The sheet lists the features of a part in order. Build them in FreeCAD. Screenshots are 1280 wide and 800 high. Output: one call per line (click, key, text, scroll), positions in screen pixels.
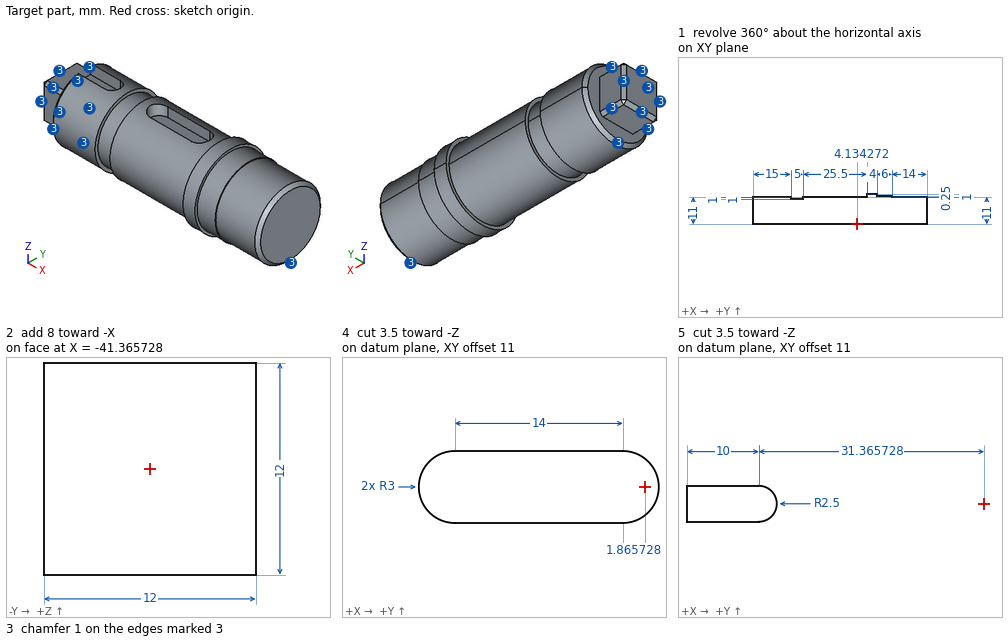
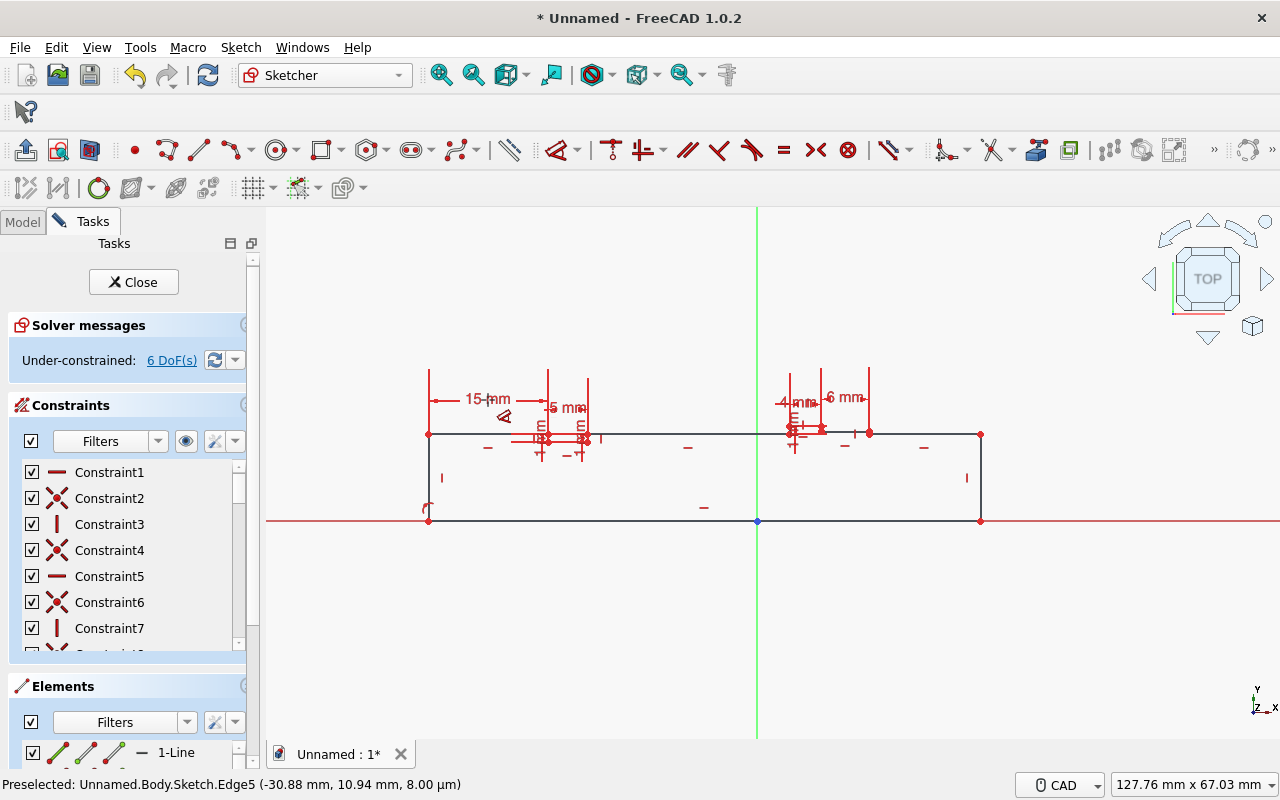
click(429, 460)
click(395, 478)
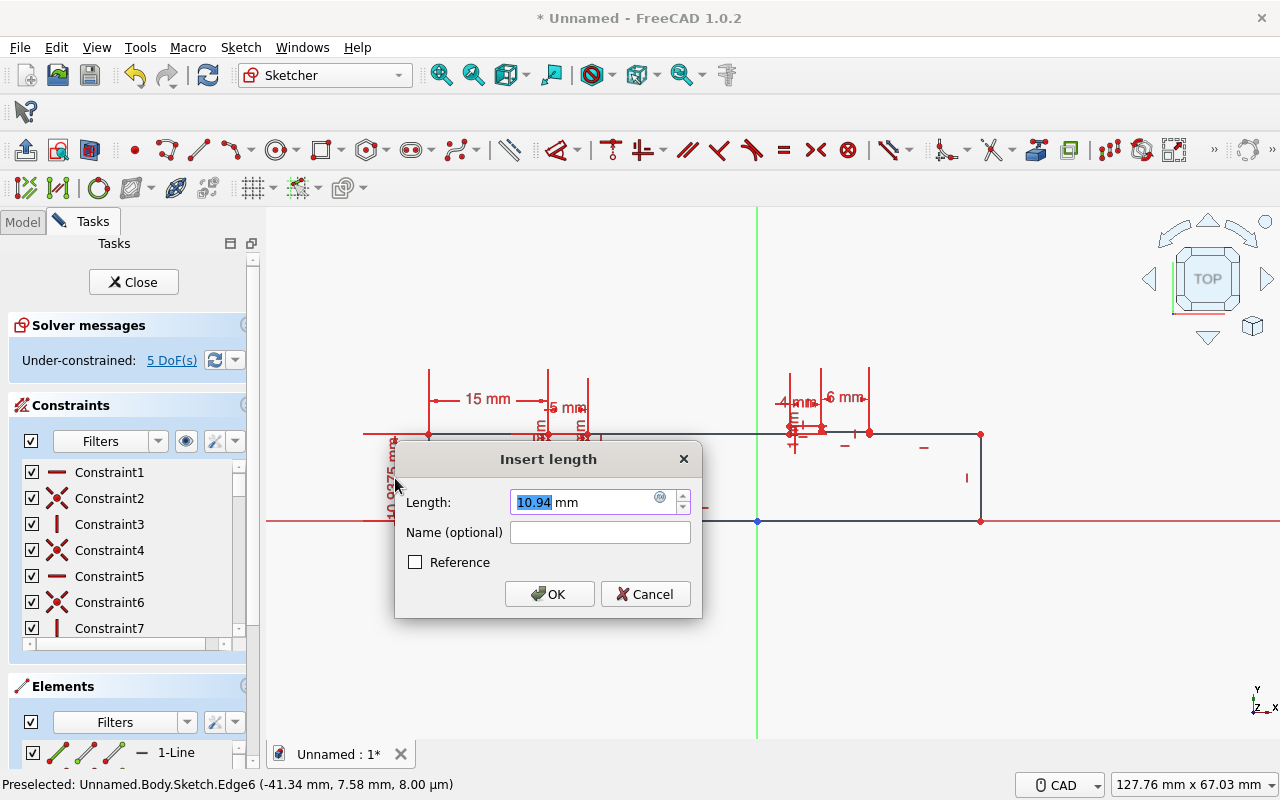
text(11)
key(Return)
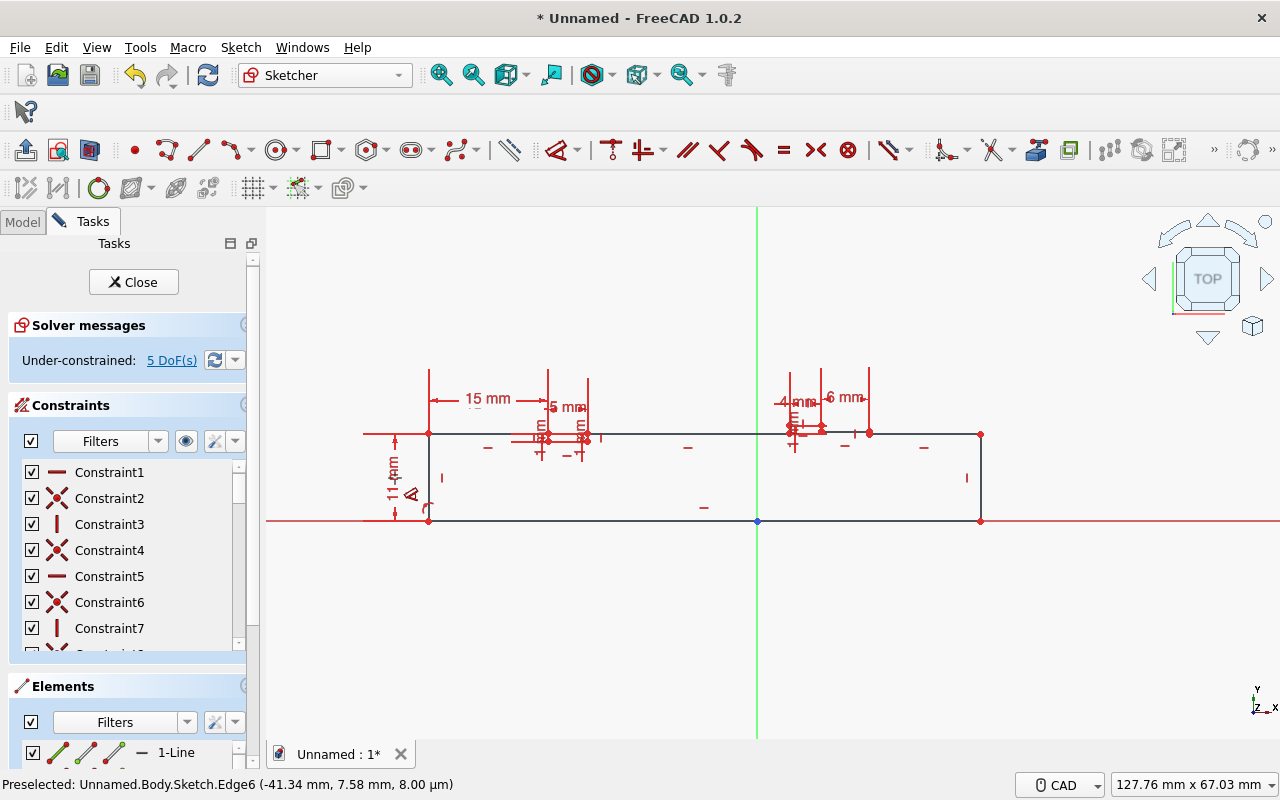
click(981, 495)
click(1015, 478)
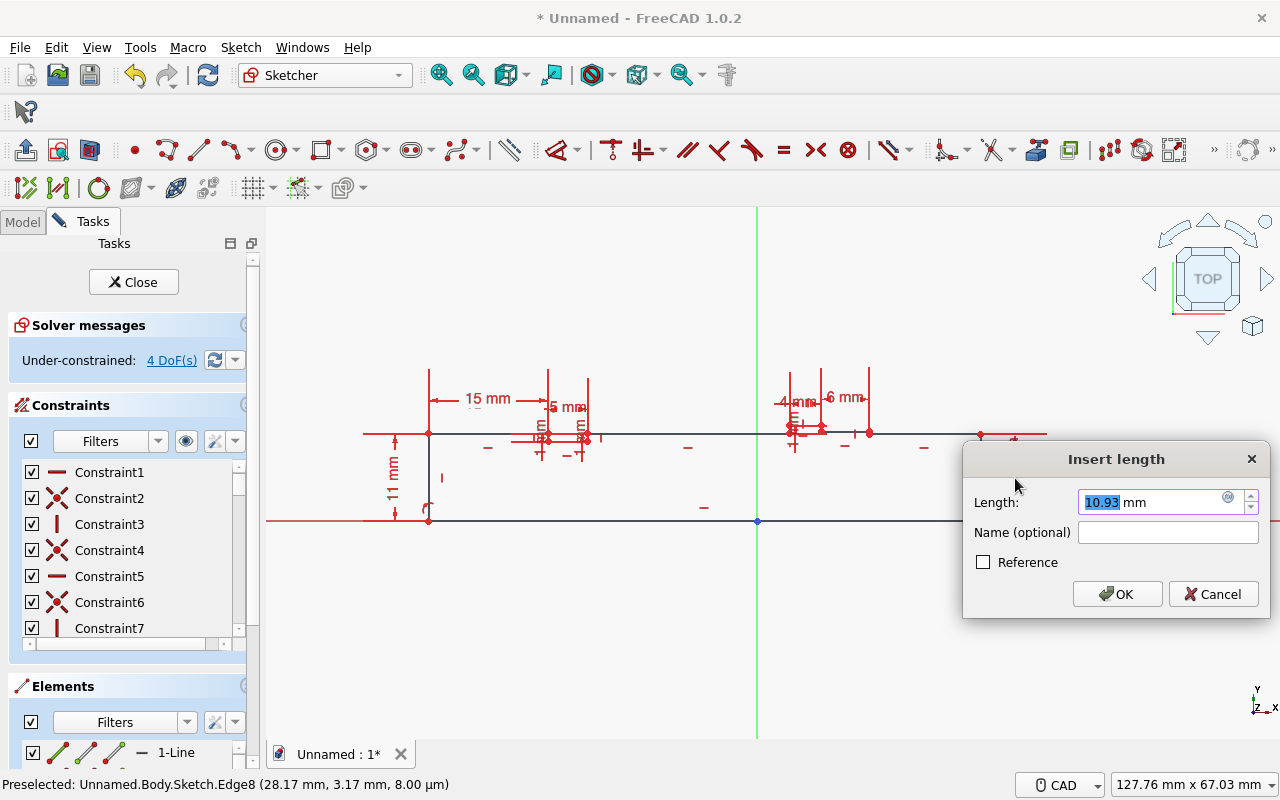
text(11)
key(Return)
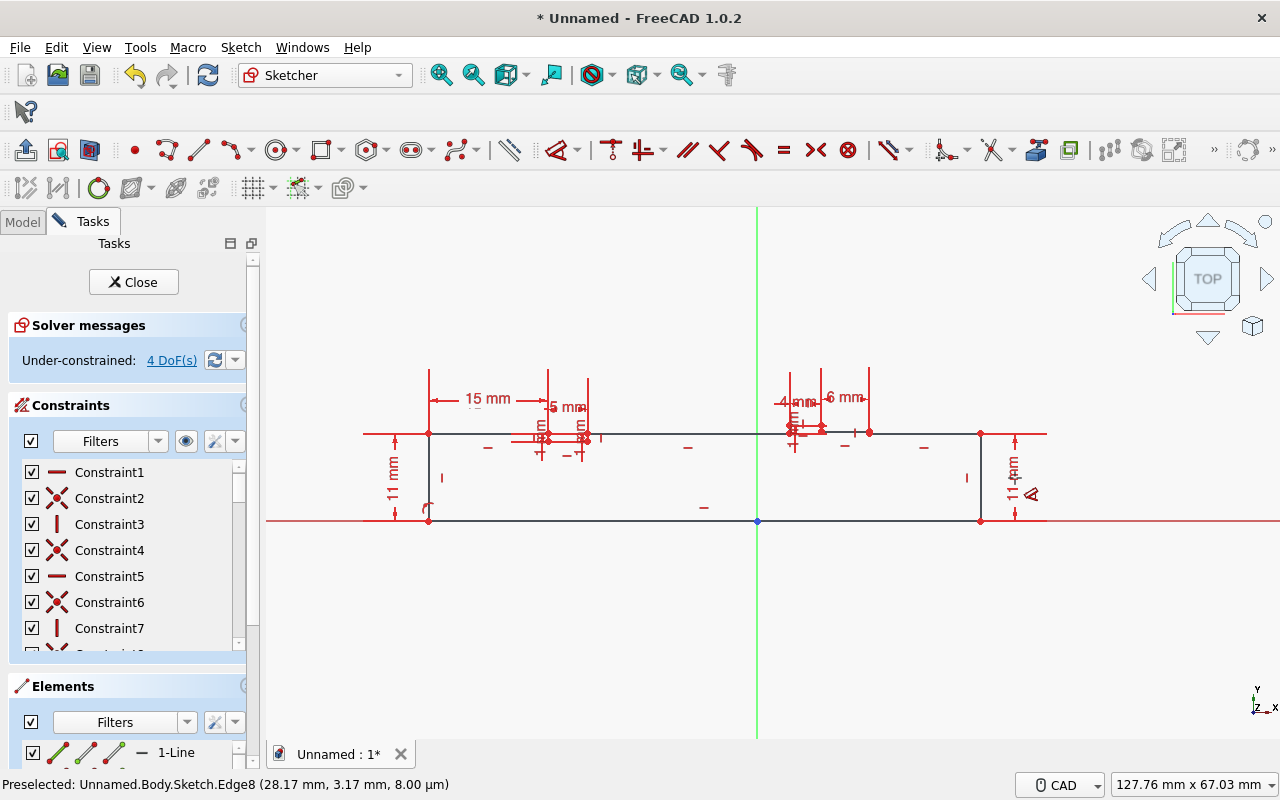
click(947, 434)
click(925, 400)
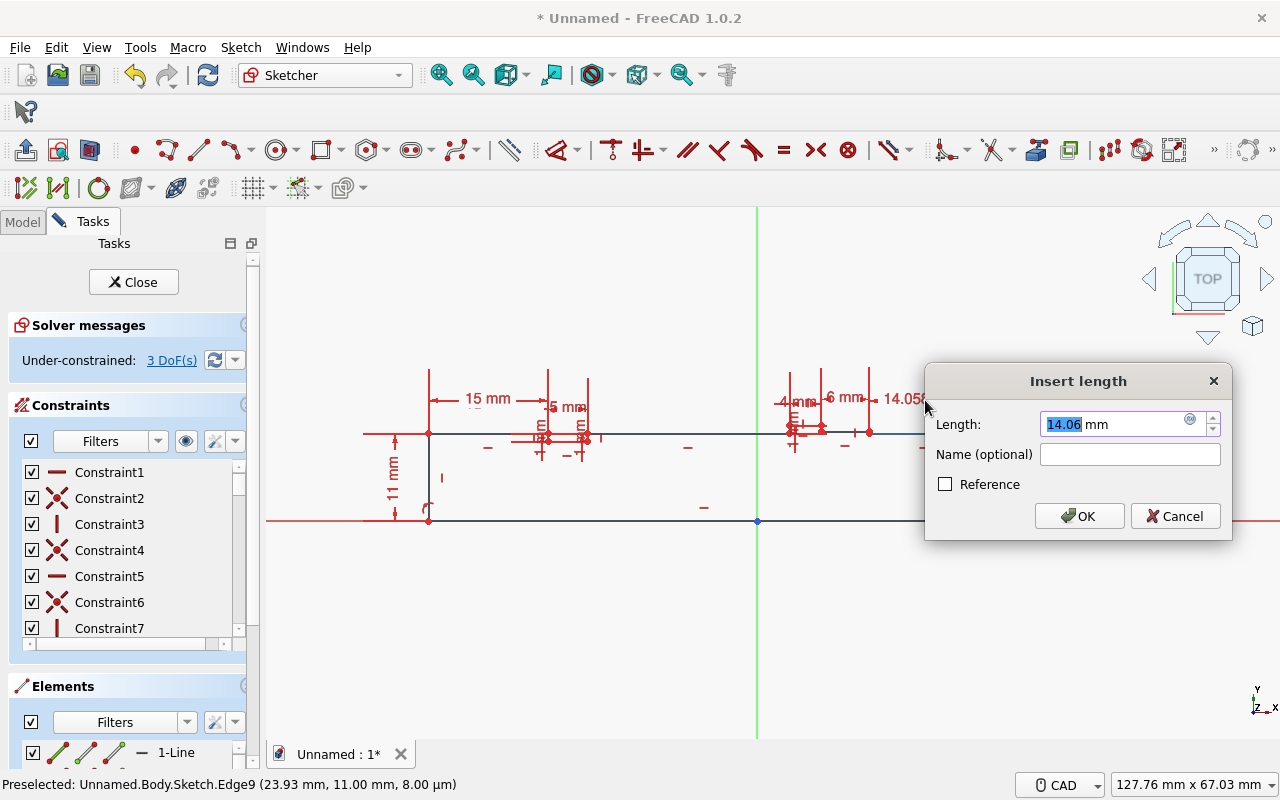
text(14)
key(Return)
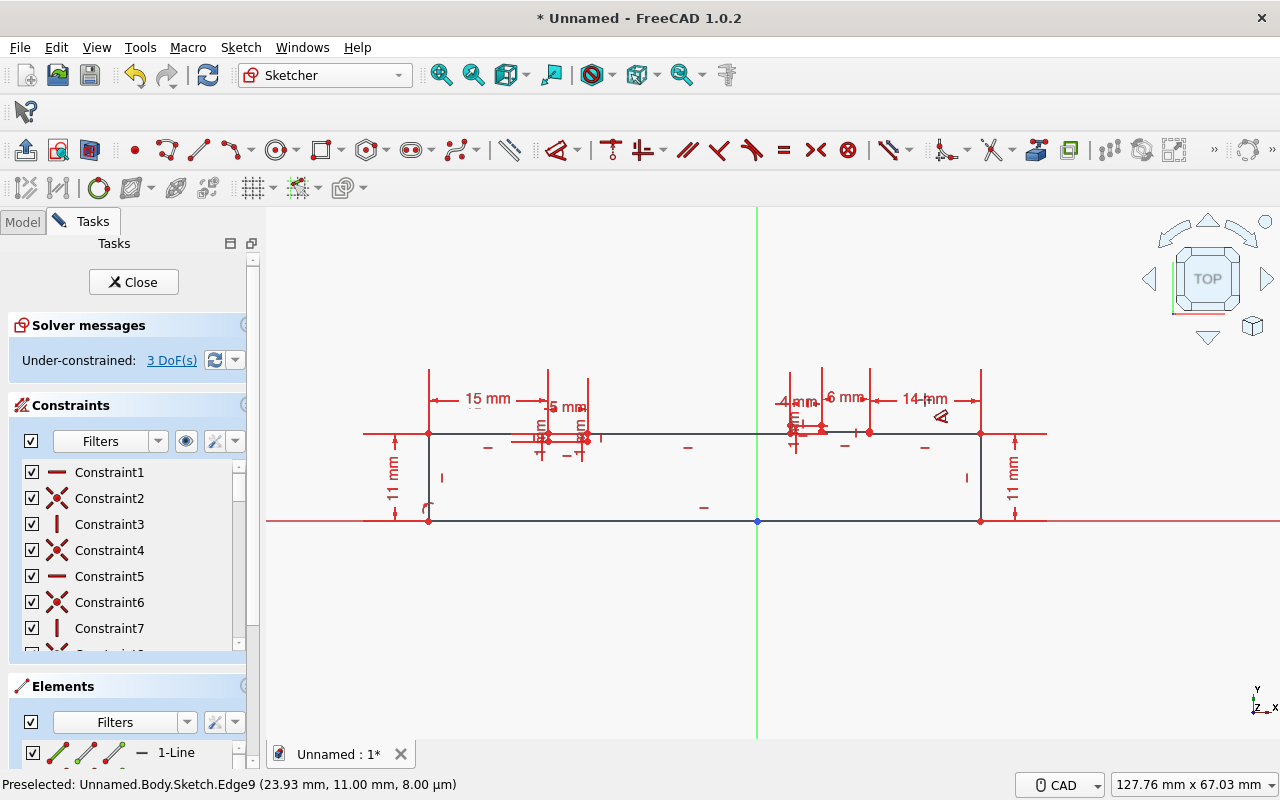
click(729, 434)
click(689, 400)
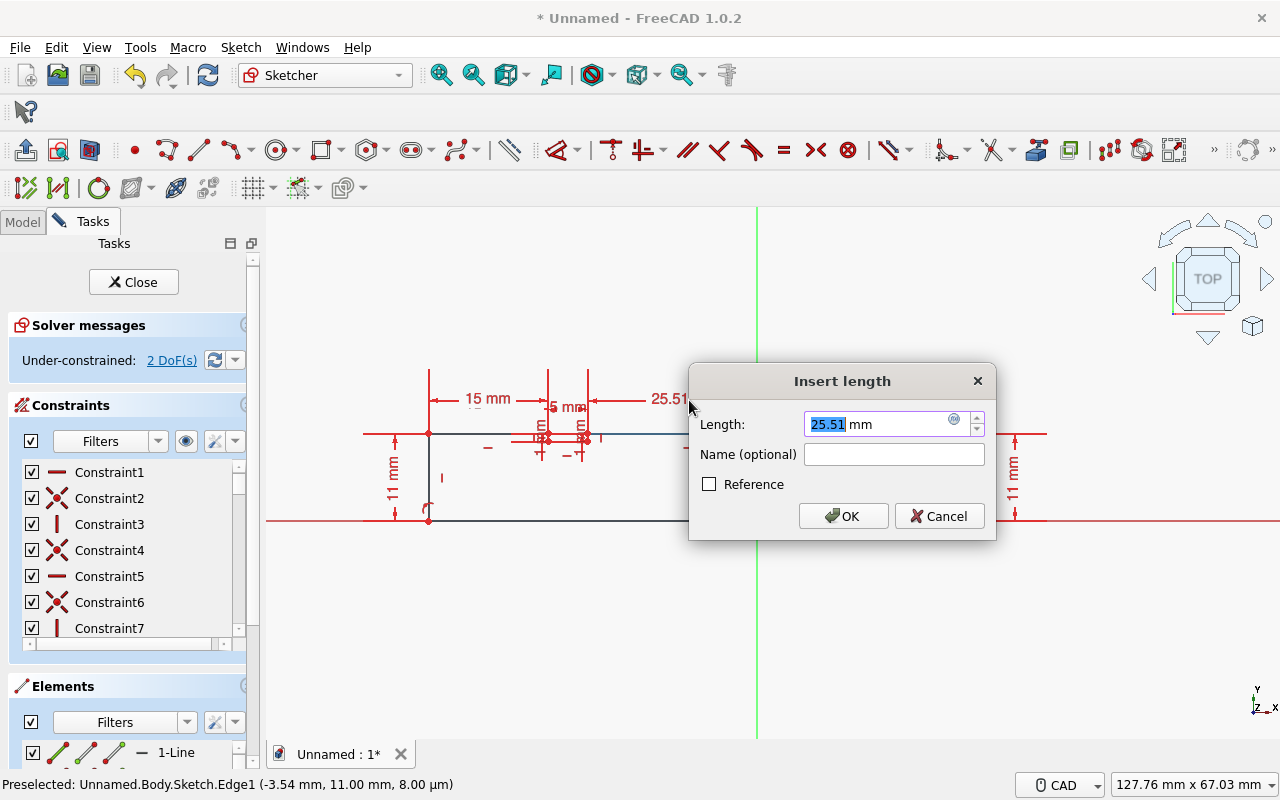
text(25.5)
key(Return)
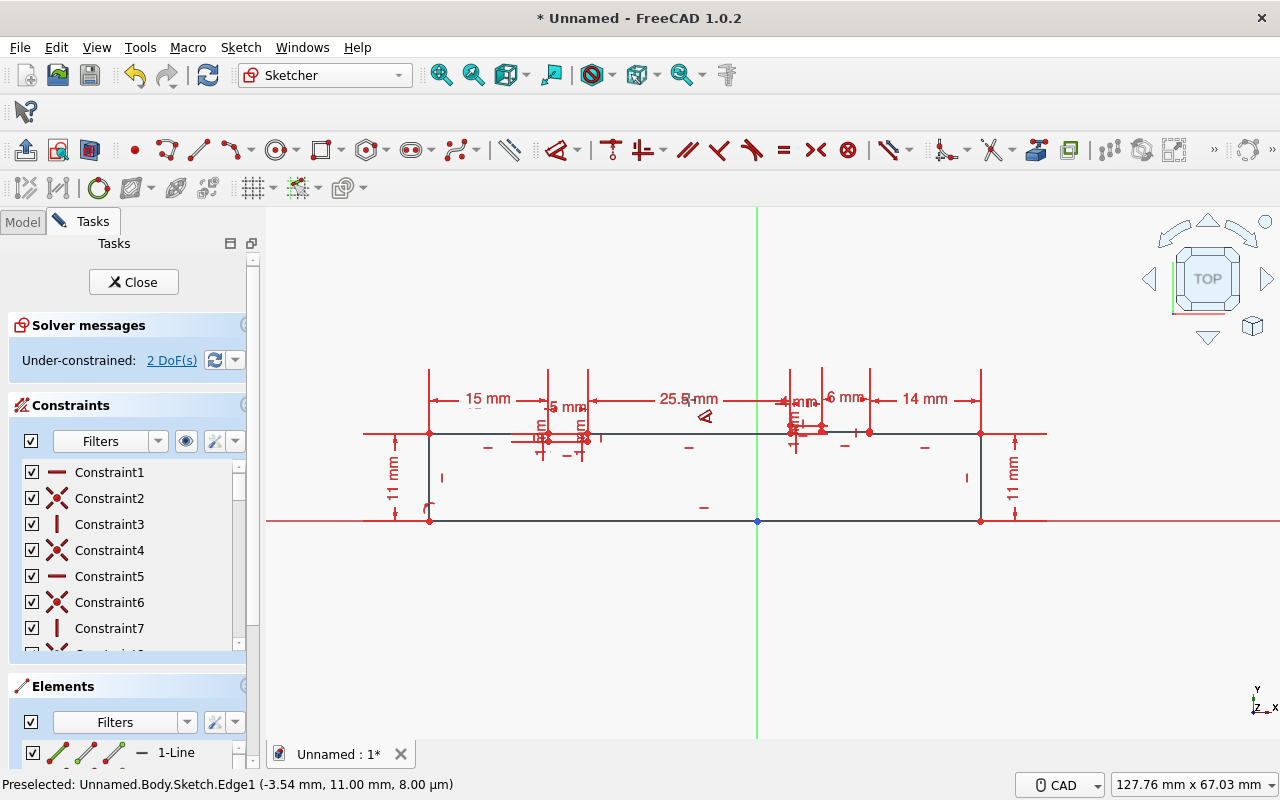
scroll(870, 433, up, 15)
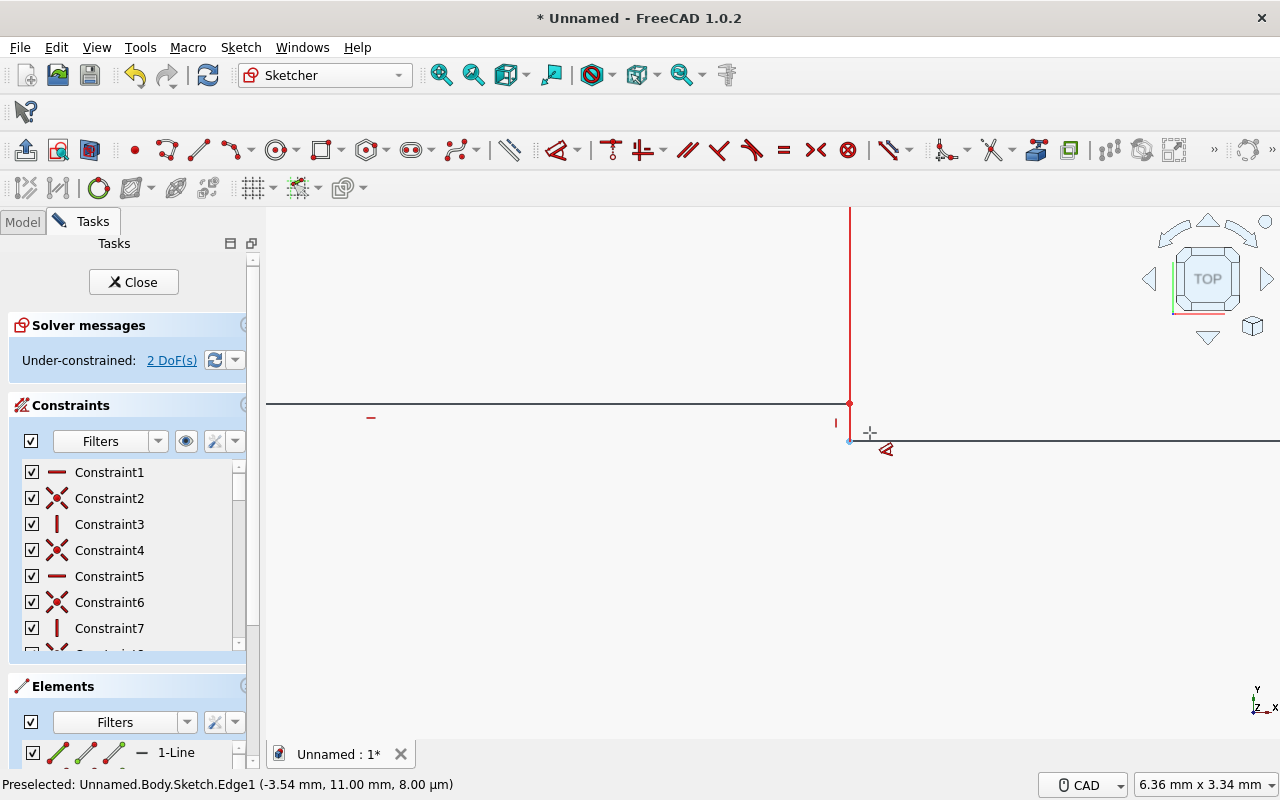
click(850, 423)
click(884, 423)